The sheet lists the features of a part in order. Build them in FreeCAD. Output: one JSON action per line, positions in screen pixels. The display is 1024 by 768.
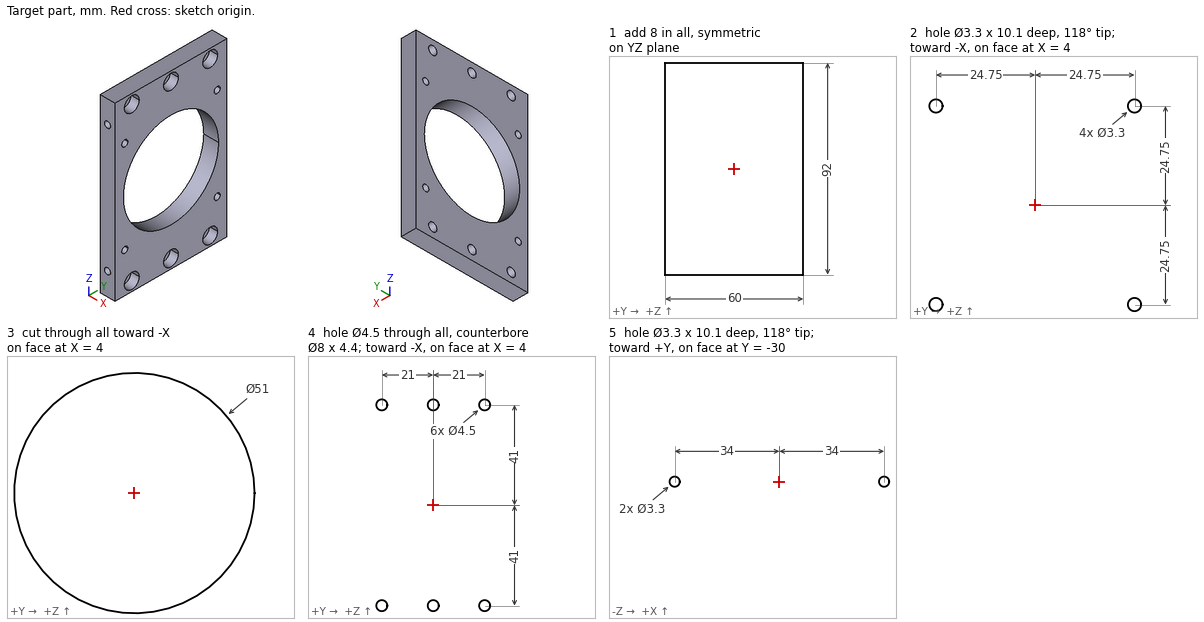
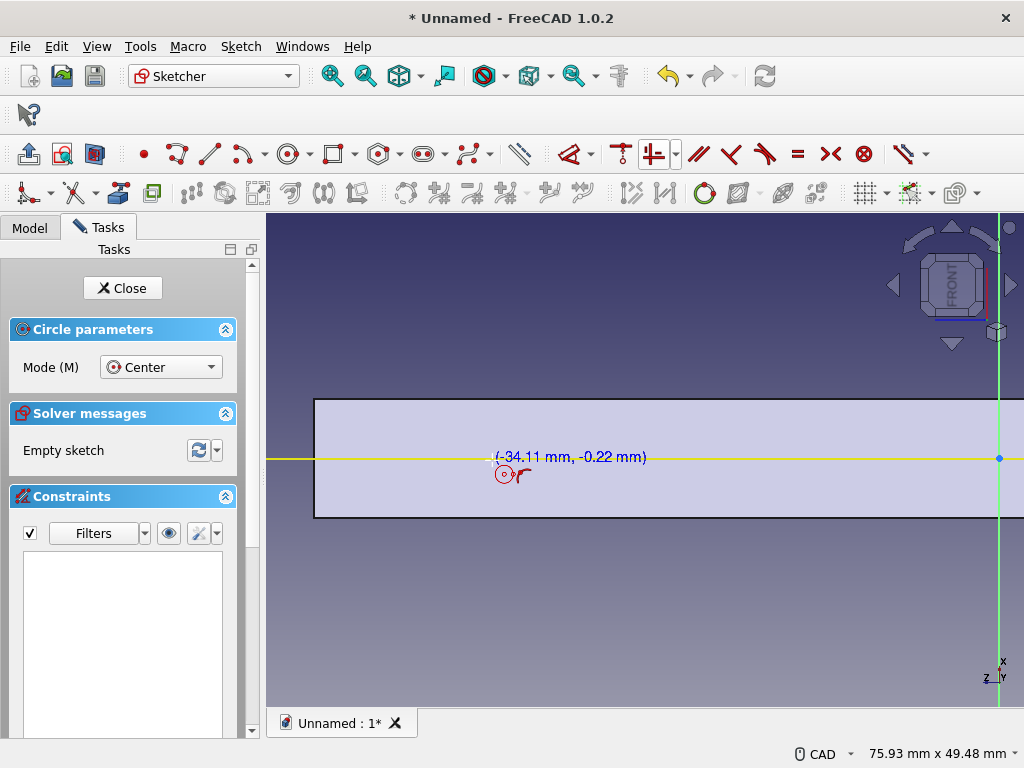
{"action": "left_click", "coordinate": [493, 459]}
{"action": "left_click", "coordinate": [510, 441]}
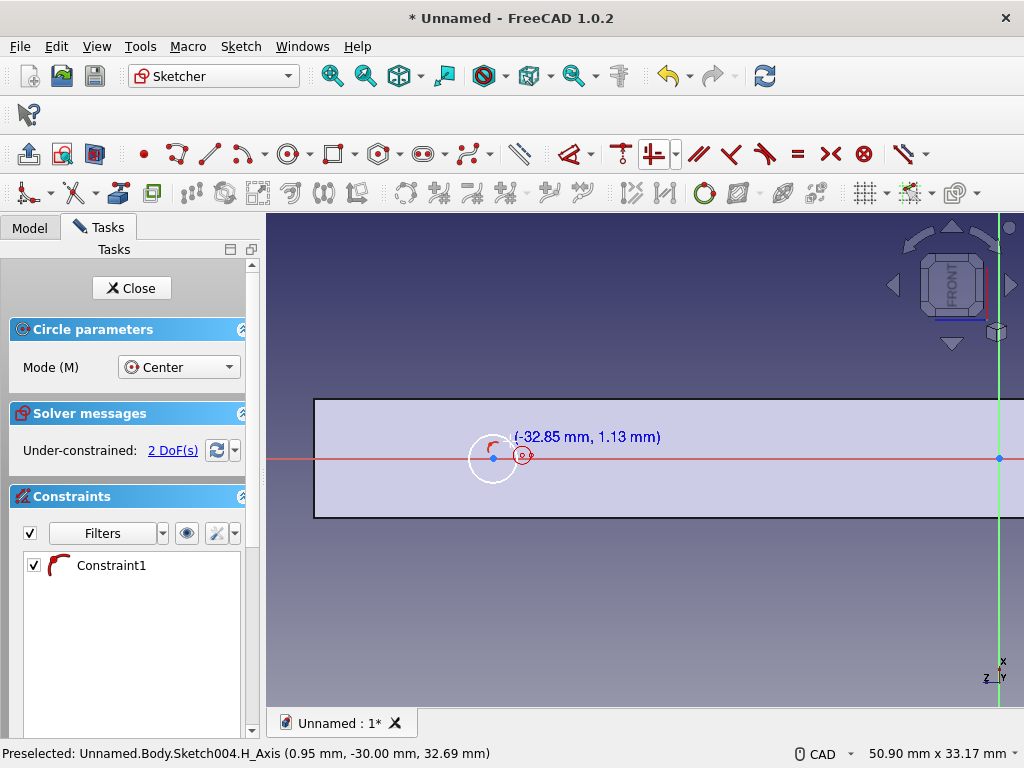
{"action": "scroll", "coordinate": [330, 461], "scroll_direction": "down", "scroll_amount": 5}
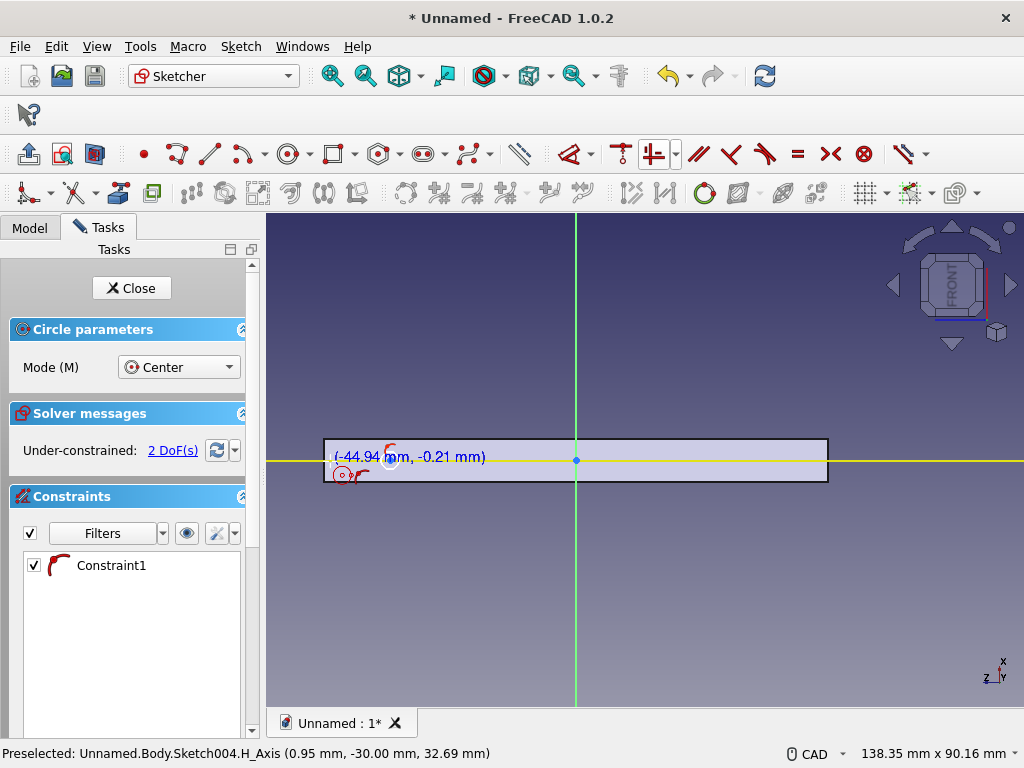
{"action": "scroll", "coordinate": [763, 461], "scroll_direction": "up", "scroll_amount": 5}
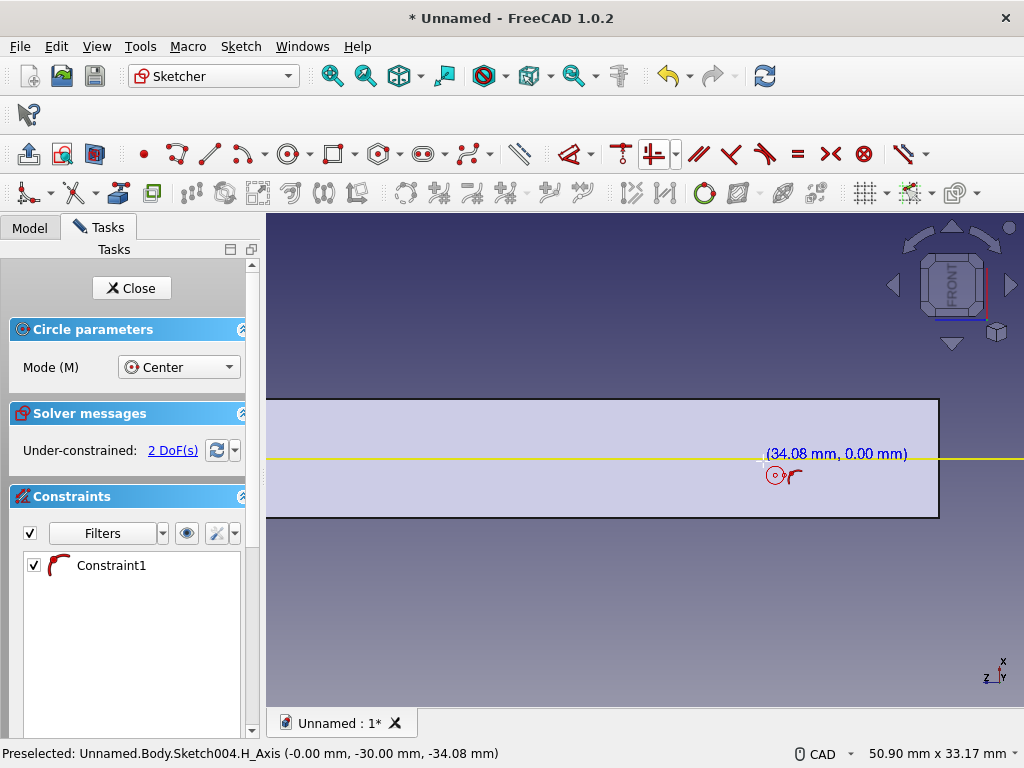
{"action": "left_click", "coordinate": [761, 459]}
{"action": "left_click", "coordinate": [778, 441]}
{"action": "key", "text": "Escape"}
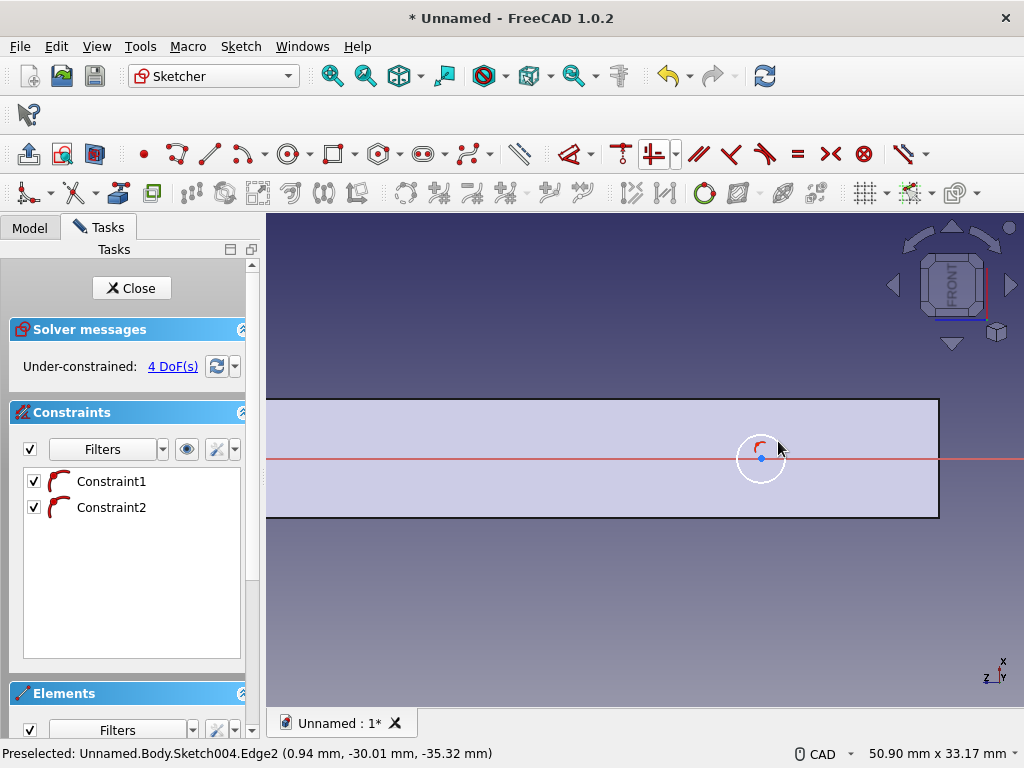
{"action": "scroll", "coordinate": [764, 461], "scroll_direction": "down", "scroll_amount": 5}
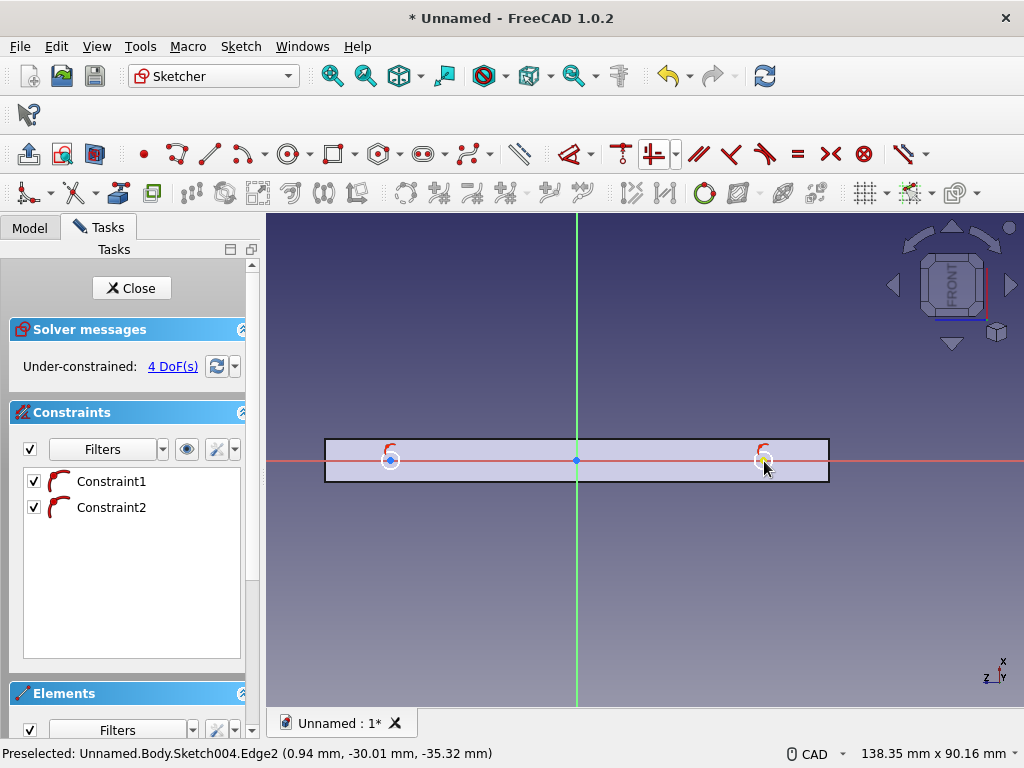
{"action": "scroll", "coordinate": [397, 454], "scroll_direction": "up", "scroll_amount": 4}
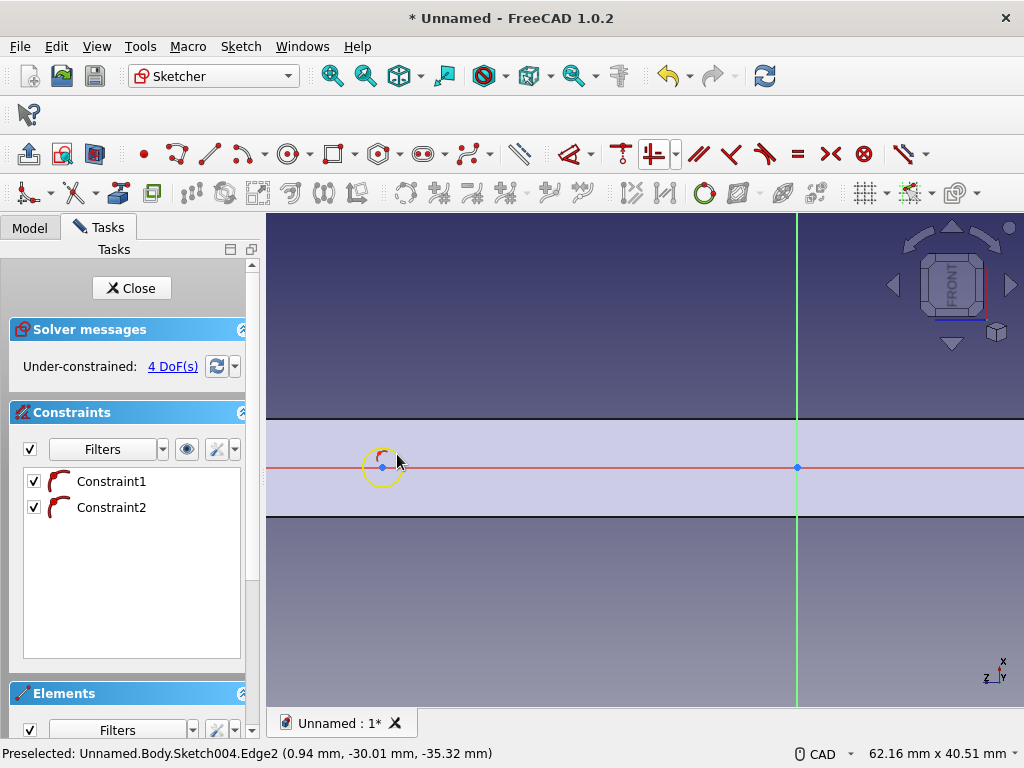
{"action": "left_click", "coordinate": [396, 454]}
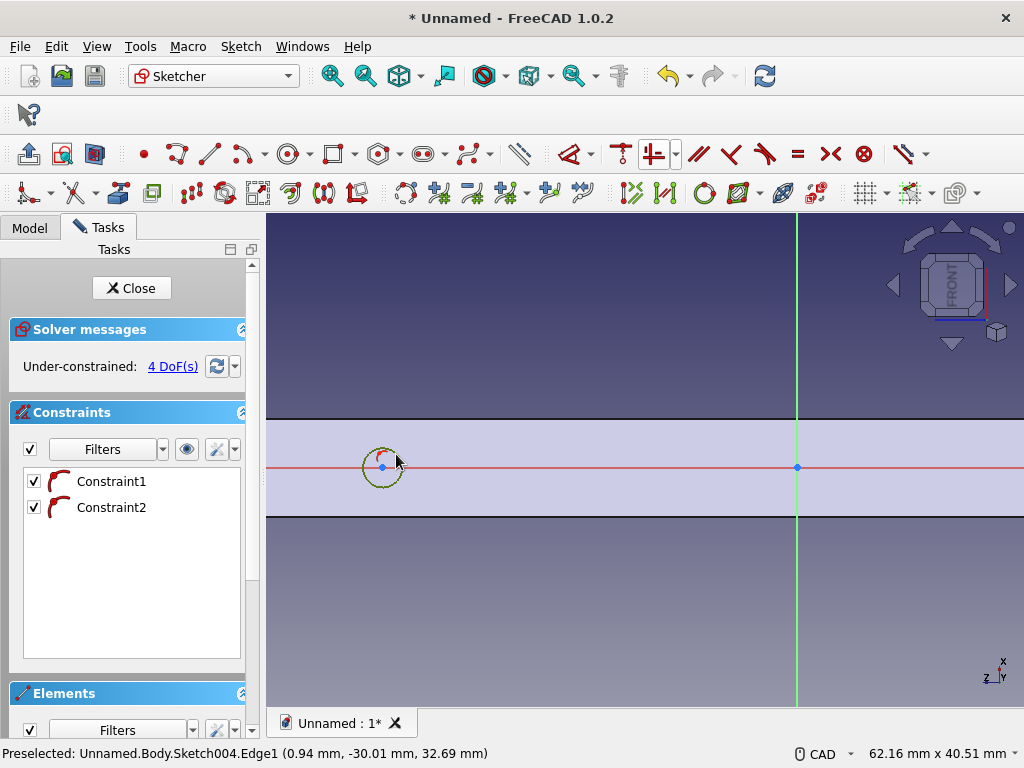
{"action": "scroll", "coordinate": [396, 454], "scroll_direction": "down", "scroll_amount": 4}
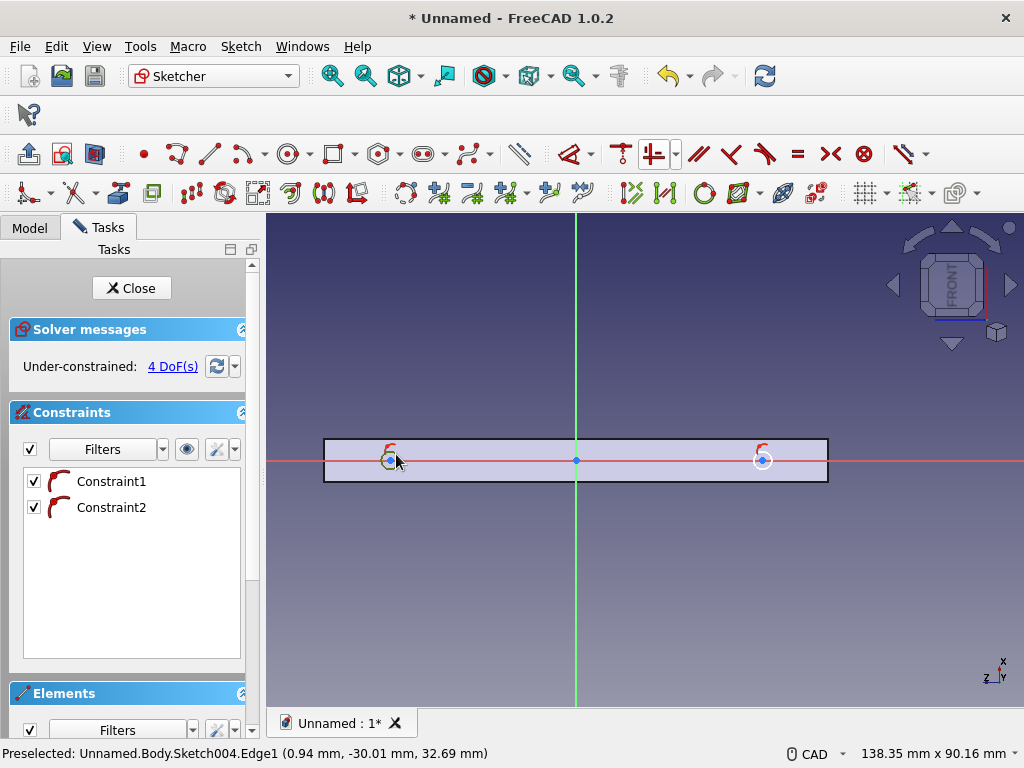
{"action": "scroll", "coordinate": [769, 454], "scroll_direction": "up", "scroll_amount": 4}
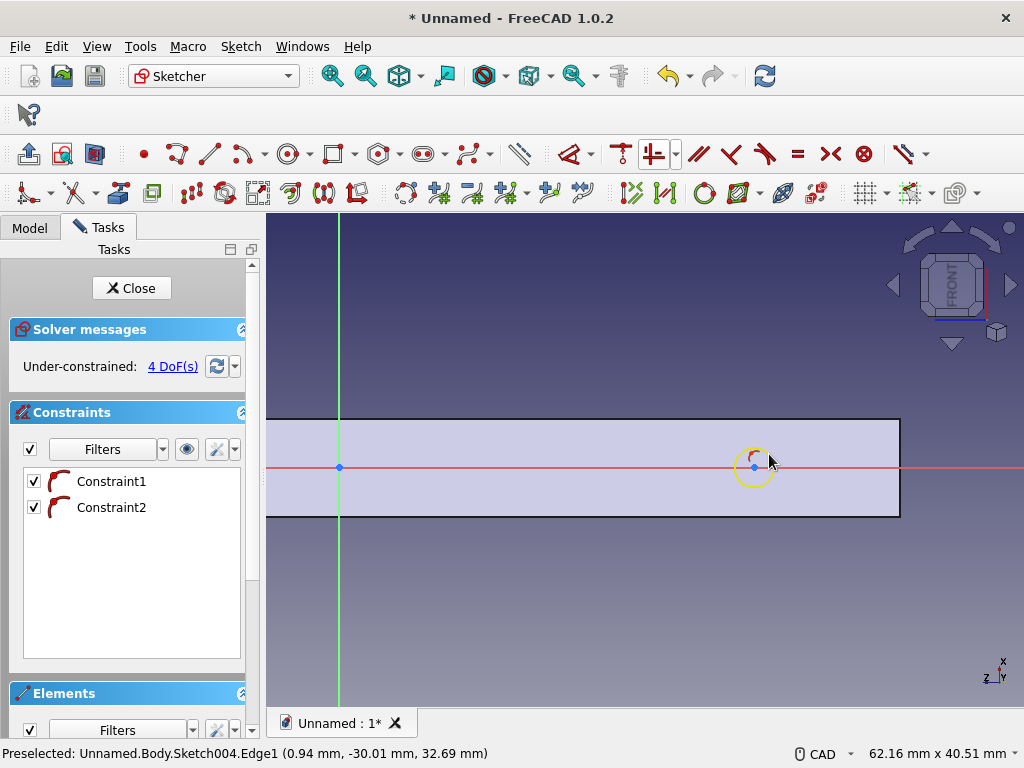
{"action": "left_click", "coordinate": [768, 454]}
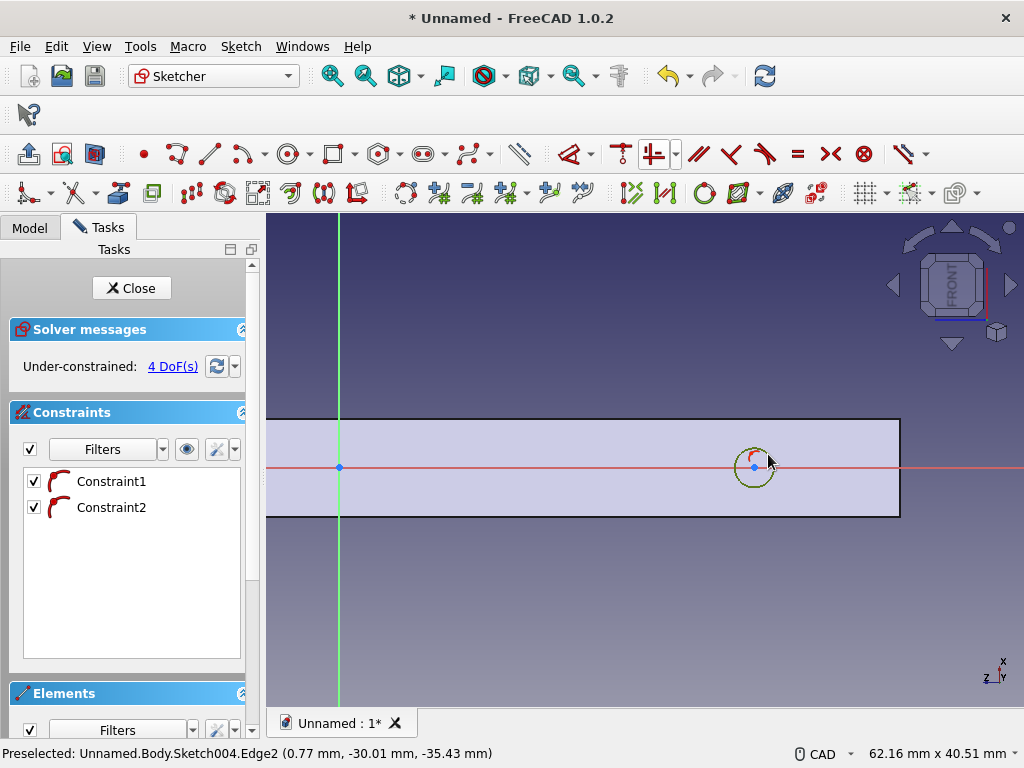
{"action": "left_click", "coordinate": [798, 154]}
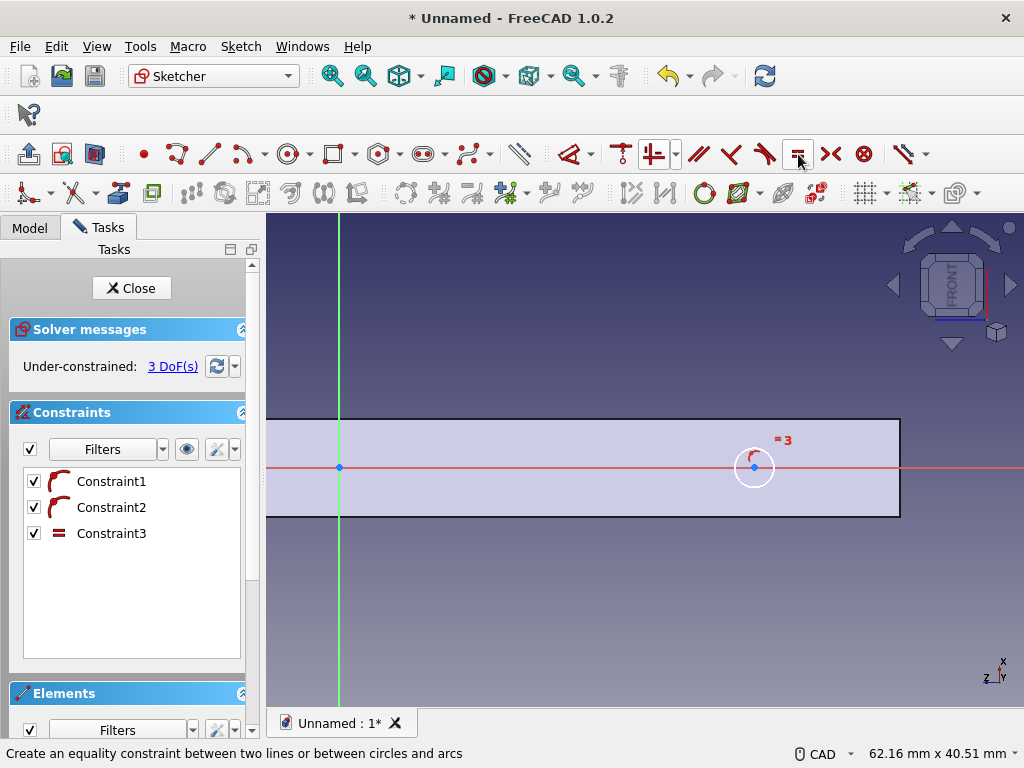
{"action": "left_click", "coordinate": [568, 154]}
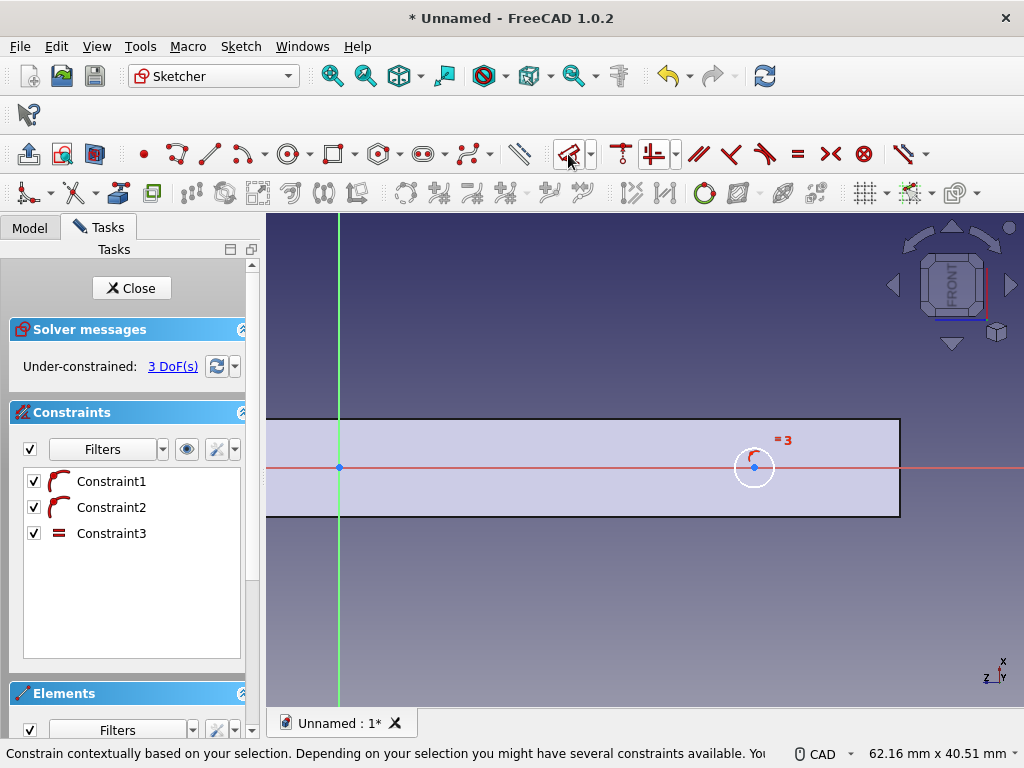
{"action": "scroll", "coordinate": [770, 454], "scroll_direction": "down", "scroll_amount": 4}